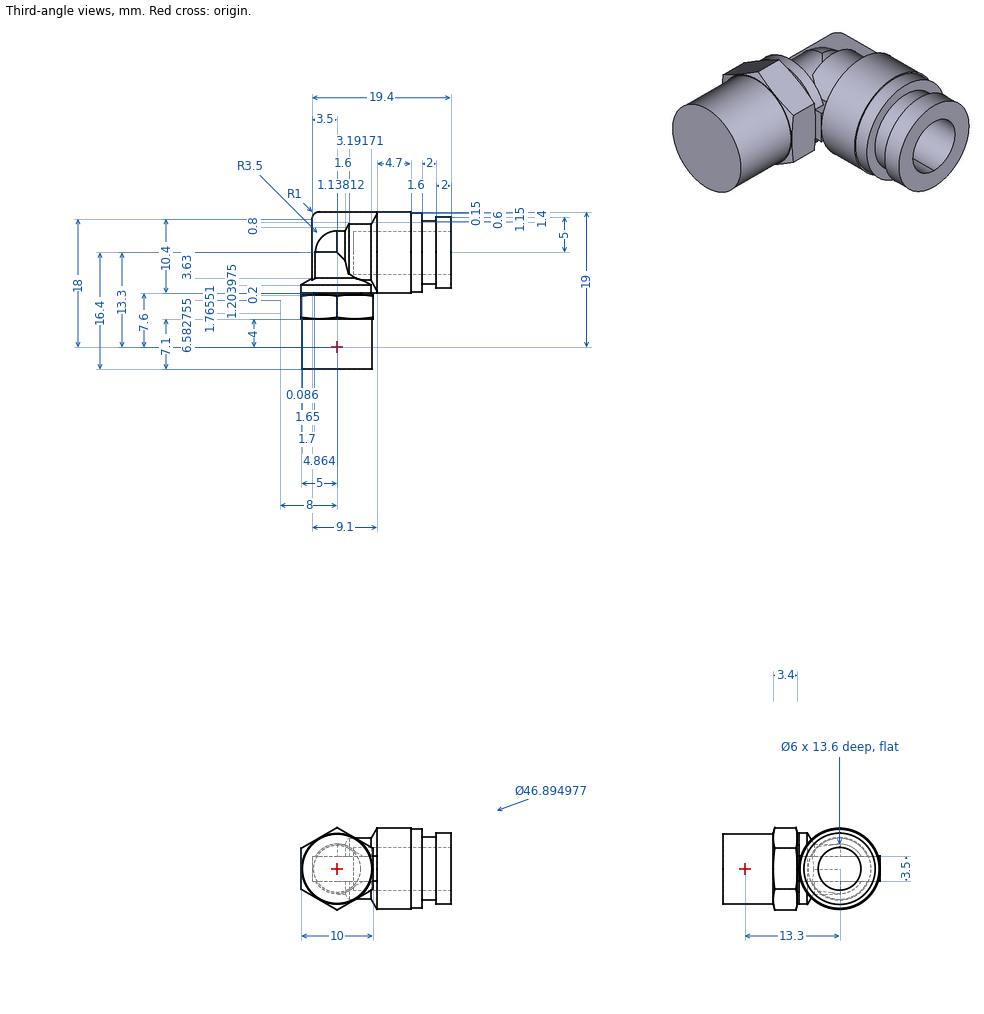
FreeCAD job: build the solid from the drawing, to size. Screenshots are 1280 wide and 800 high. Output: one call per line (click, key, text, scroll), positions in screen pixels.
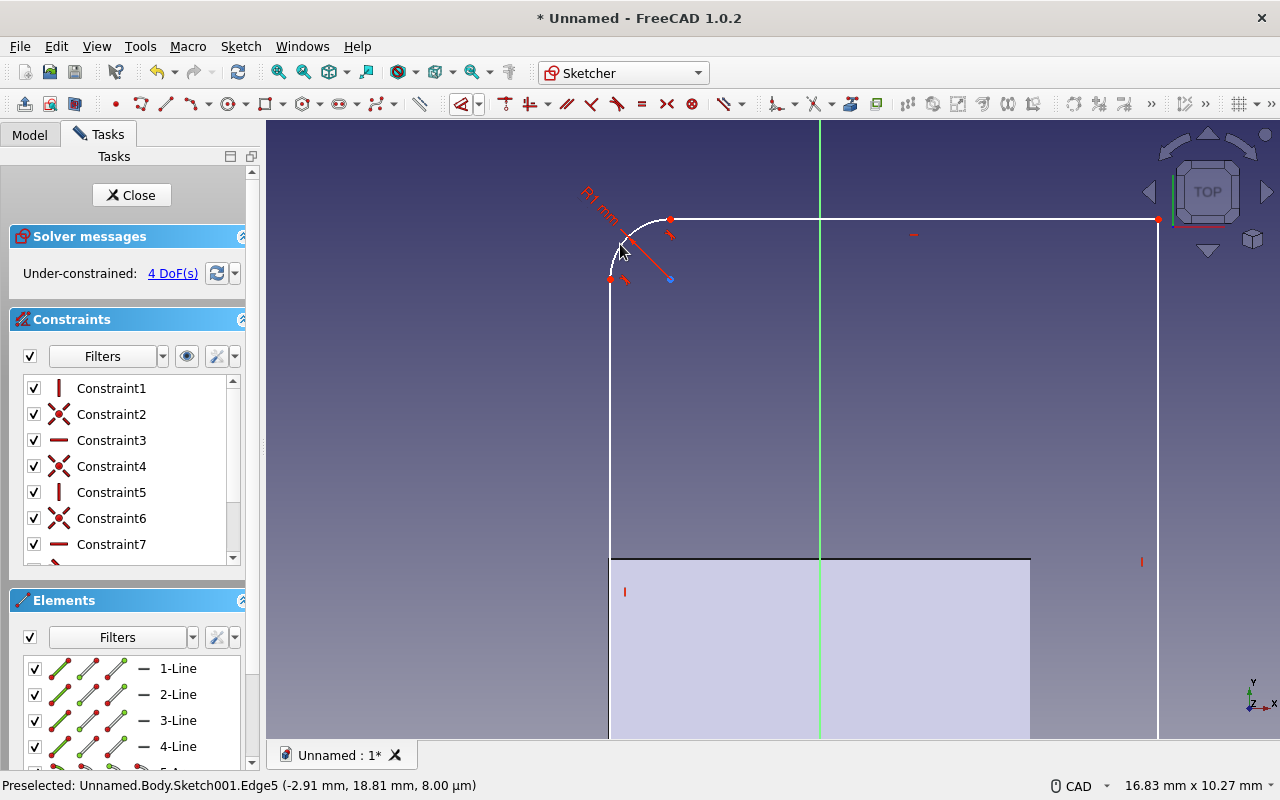
scroll(600, 221, down, 5)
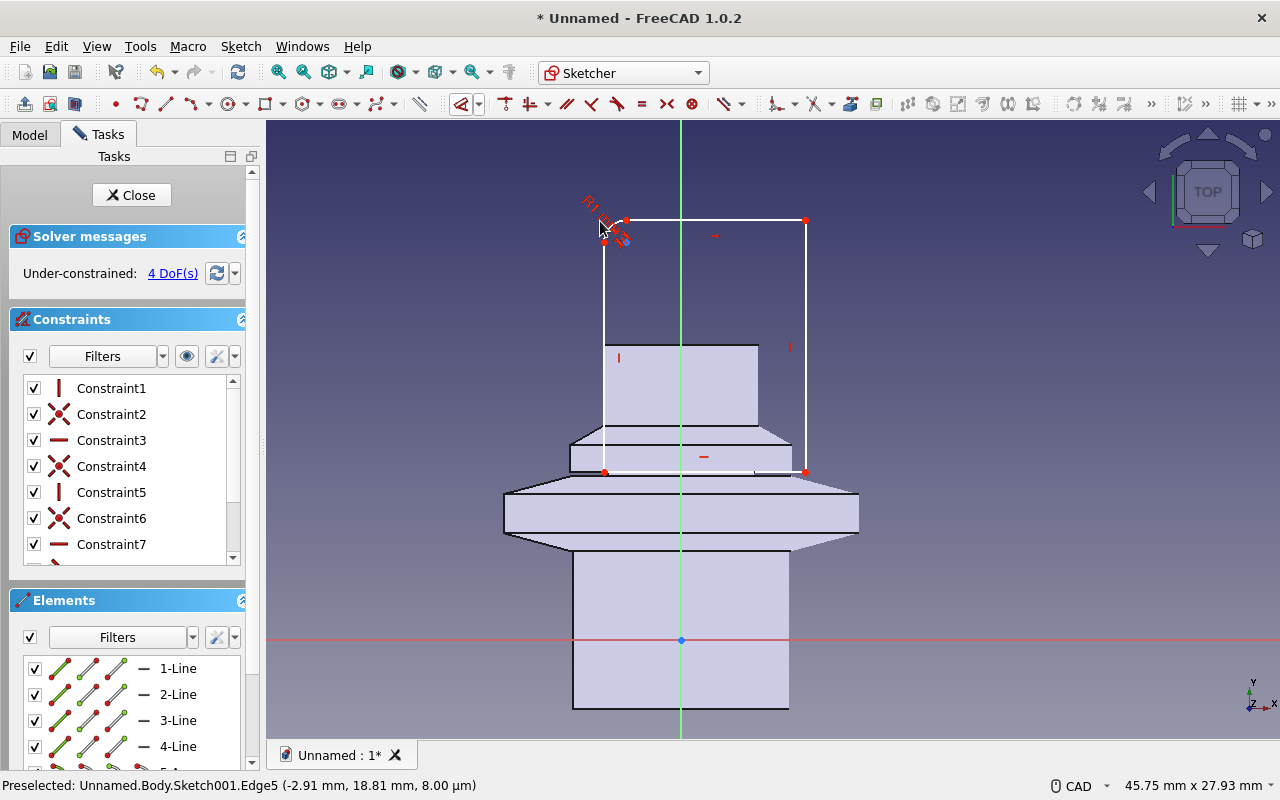
click(665, 472)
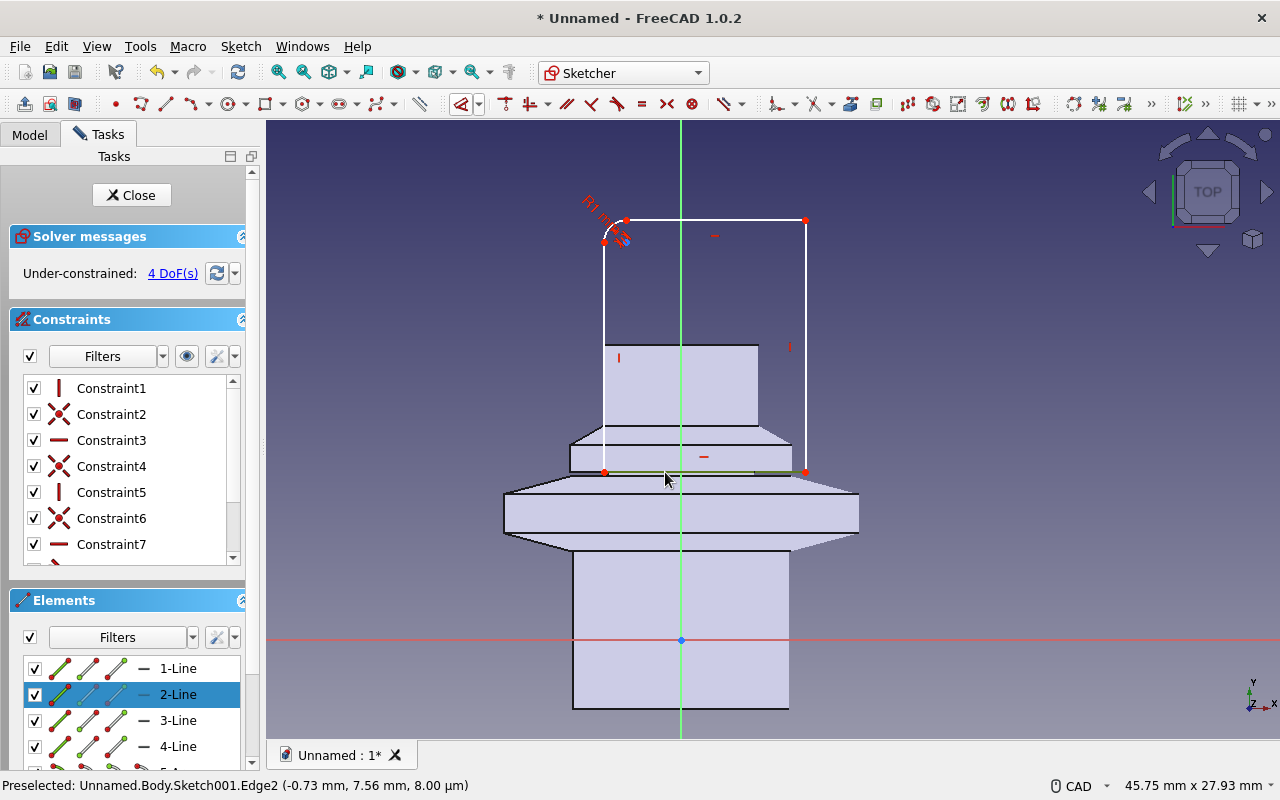
key(l)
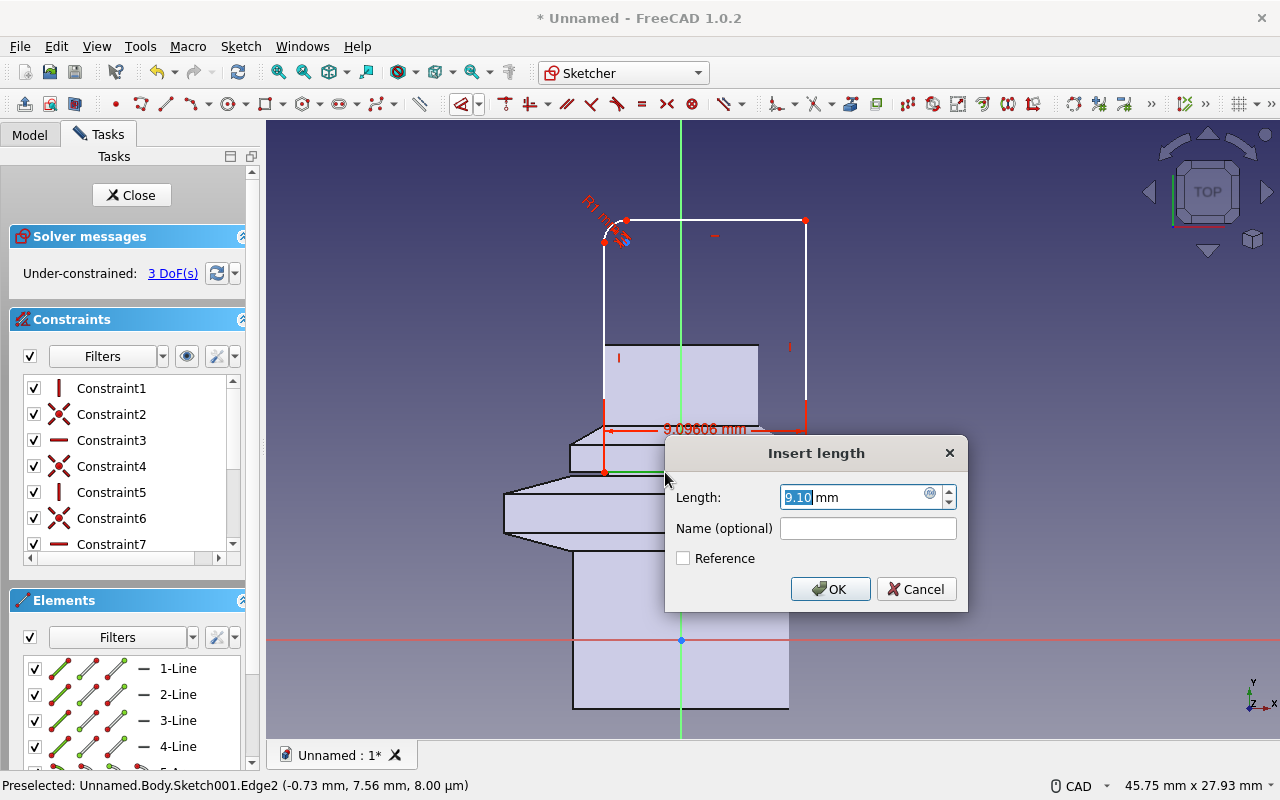
text(9.1)
key(Return)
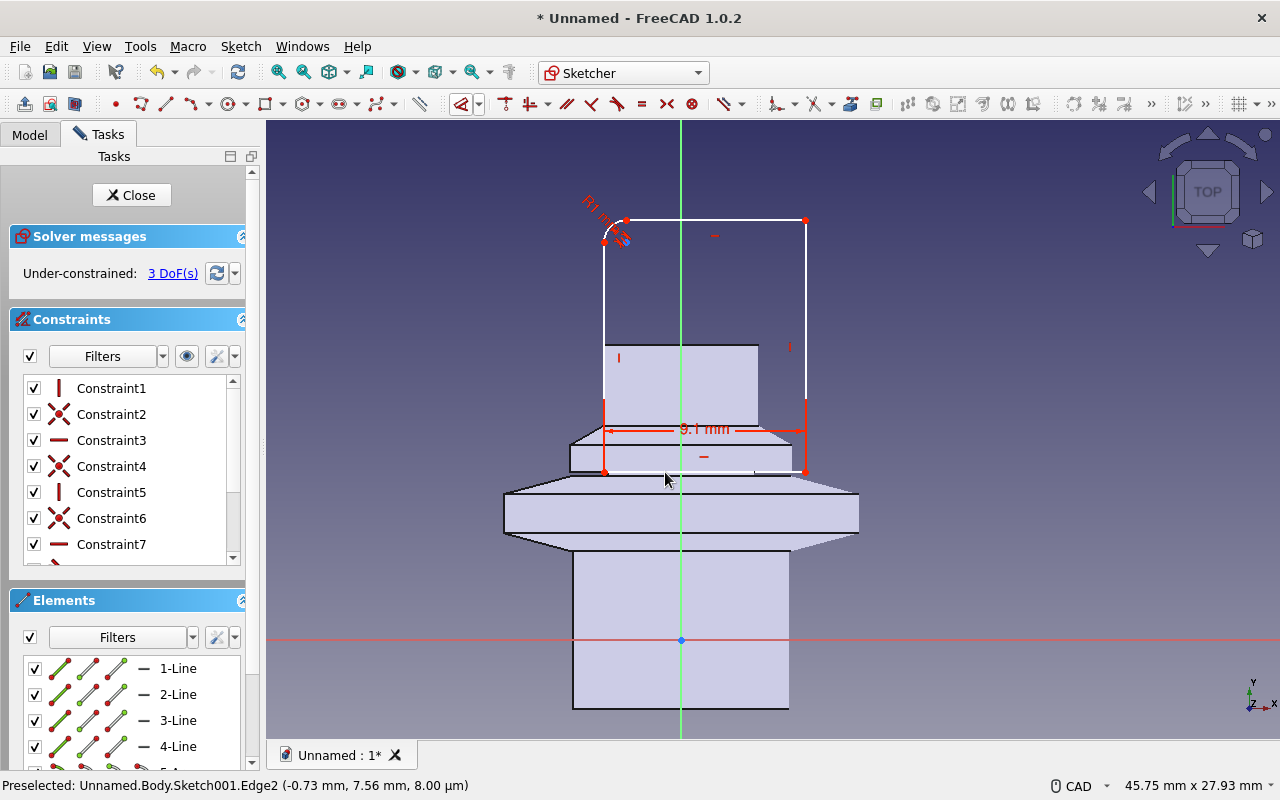
click(604, 243)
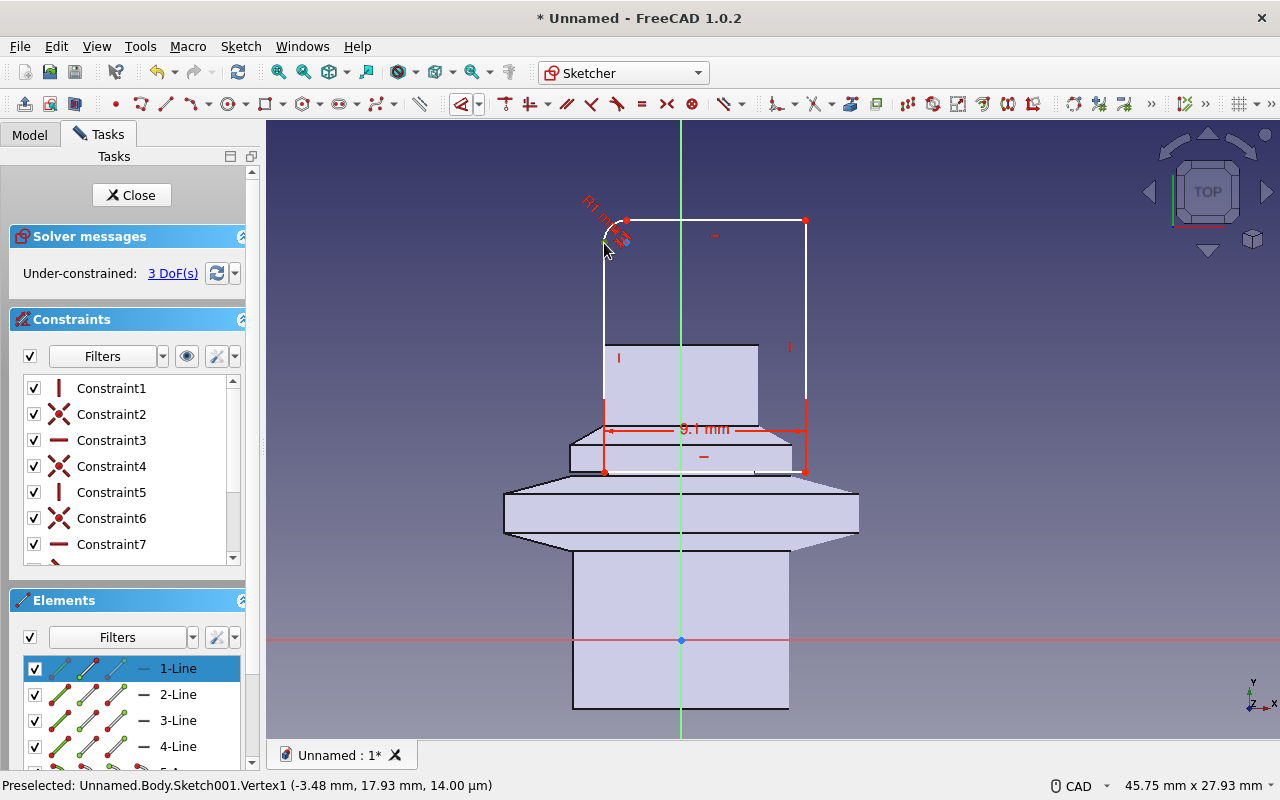
key(i)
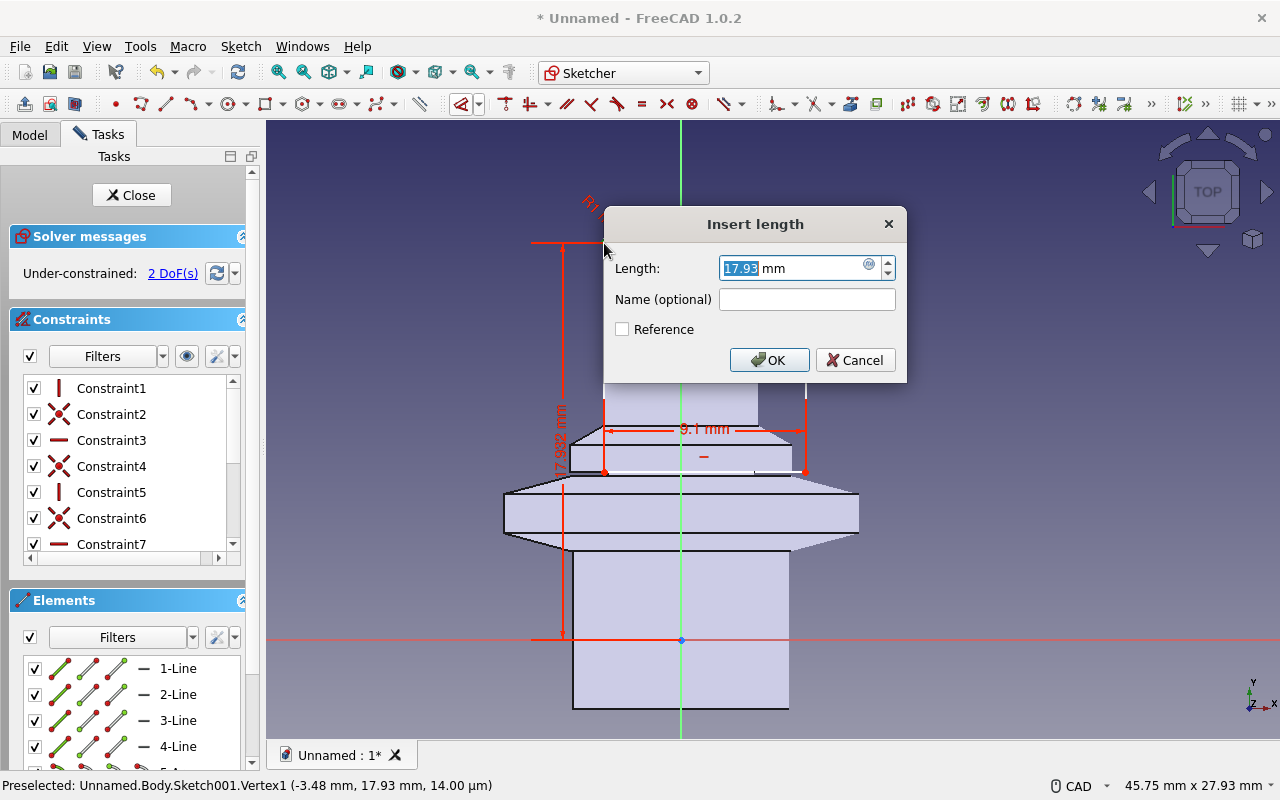
text(18)
key(Return)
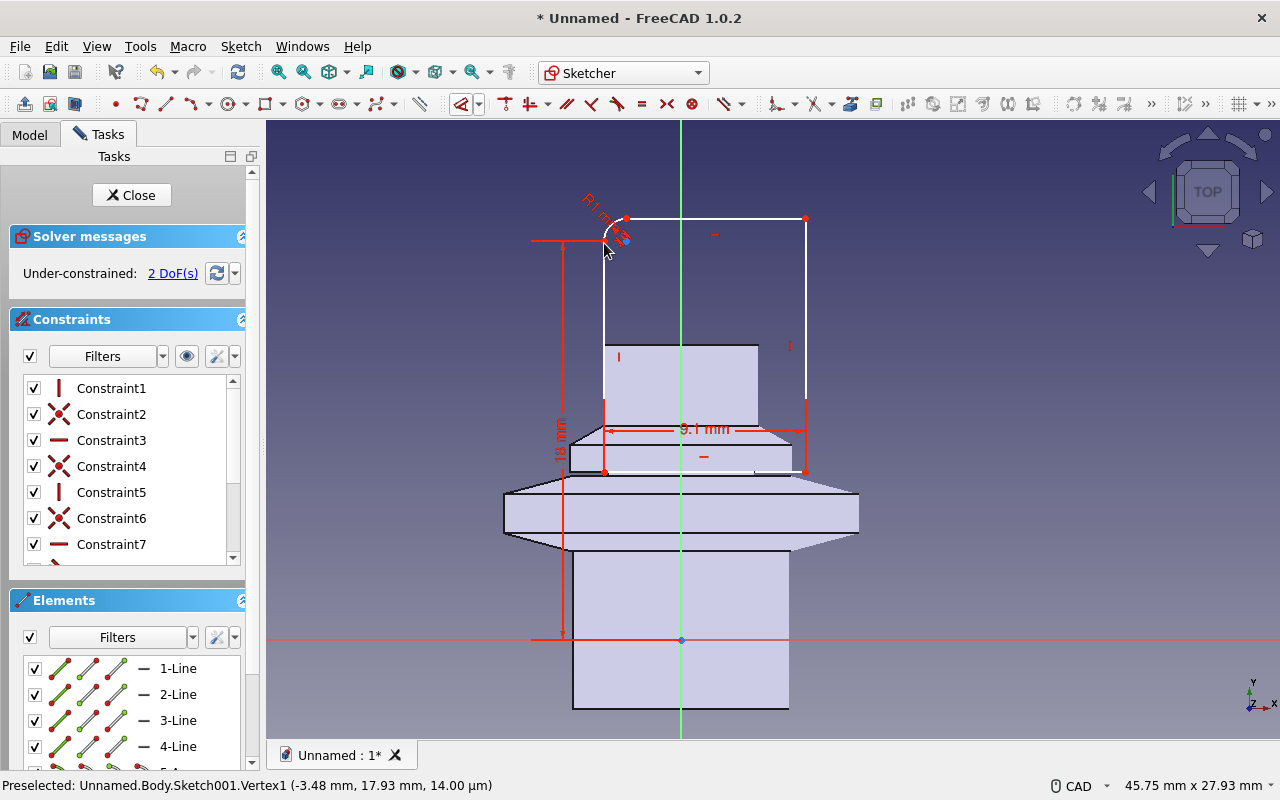
click(604, 311)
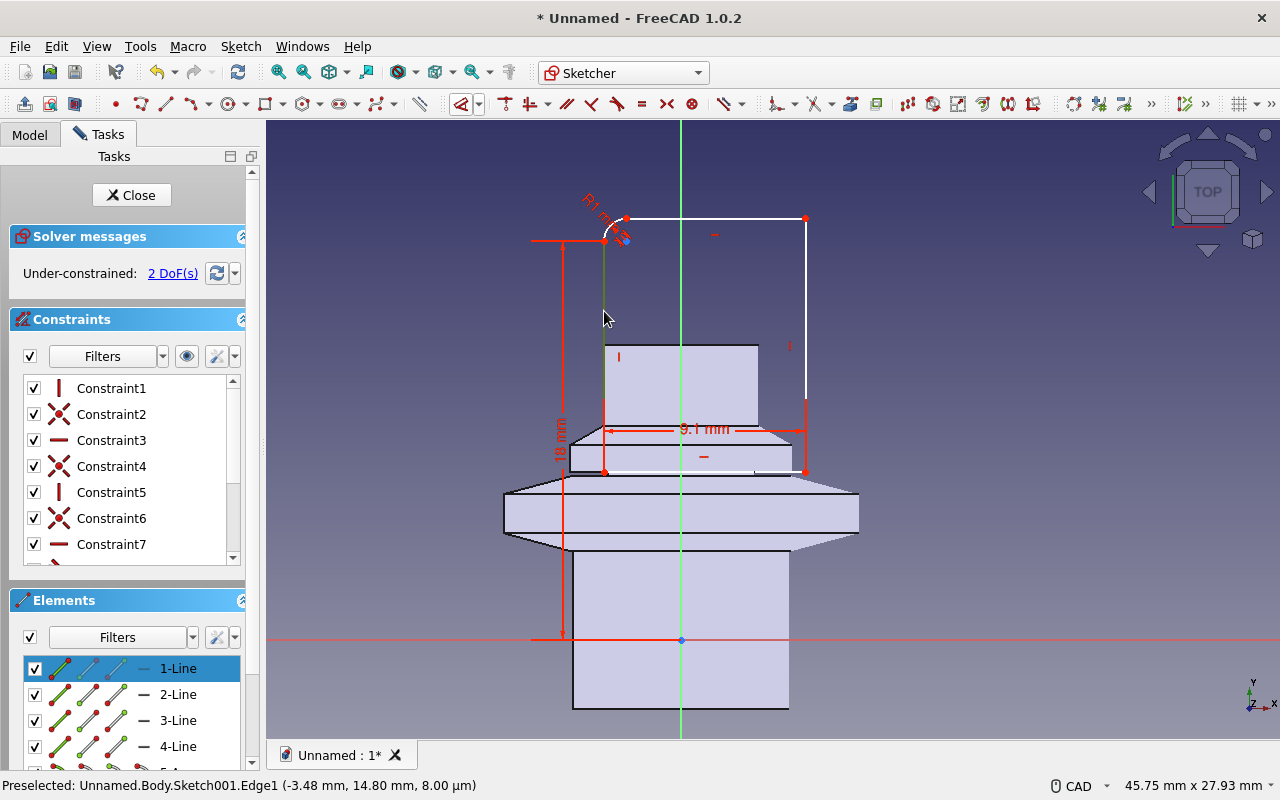
key(i)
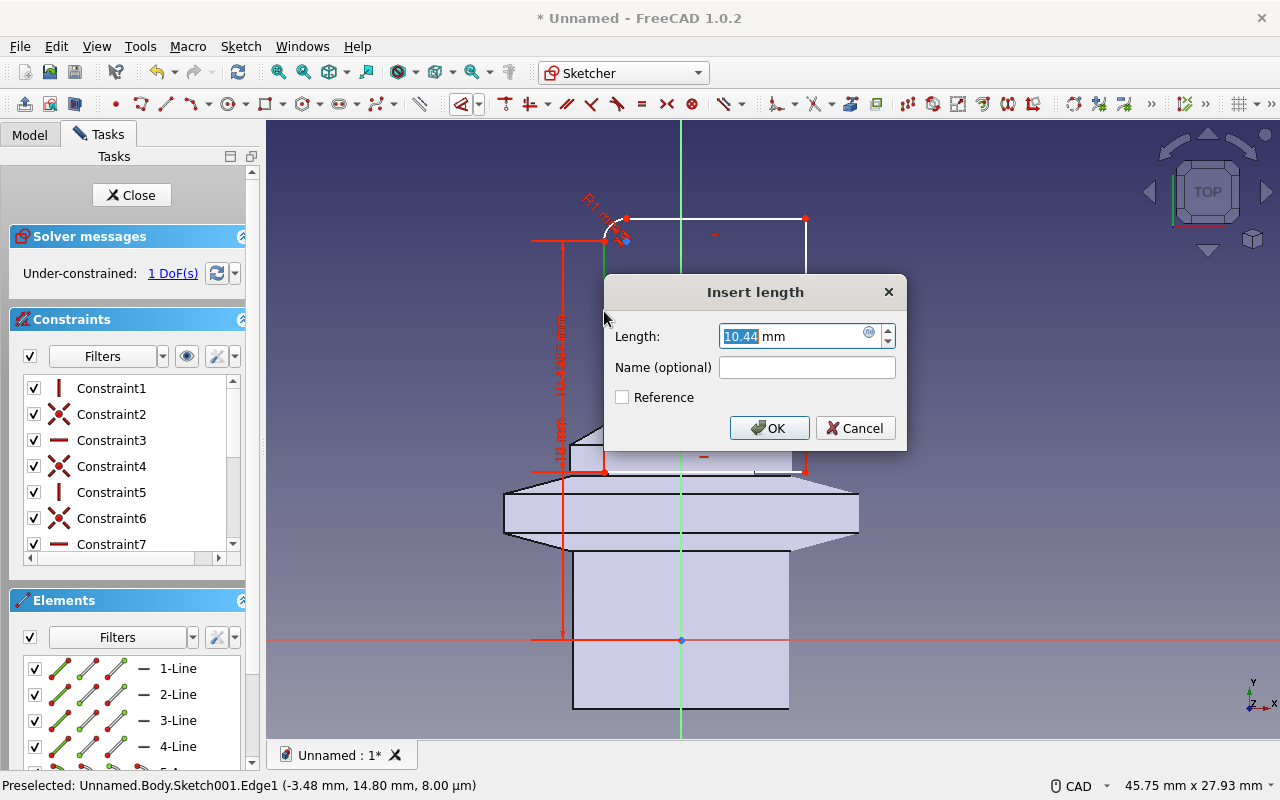
text(10.4)
key(Return)